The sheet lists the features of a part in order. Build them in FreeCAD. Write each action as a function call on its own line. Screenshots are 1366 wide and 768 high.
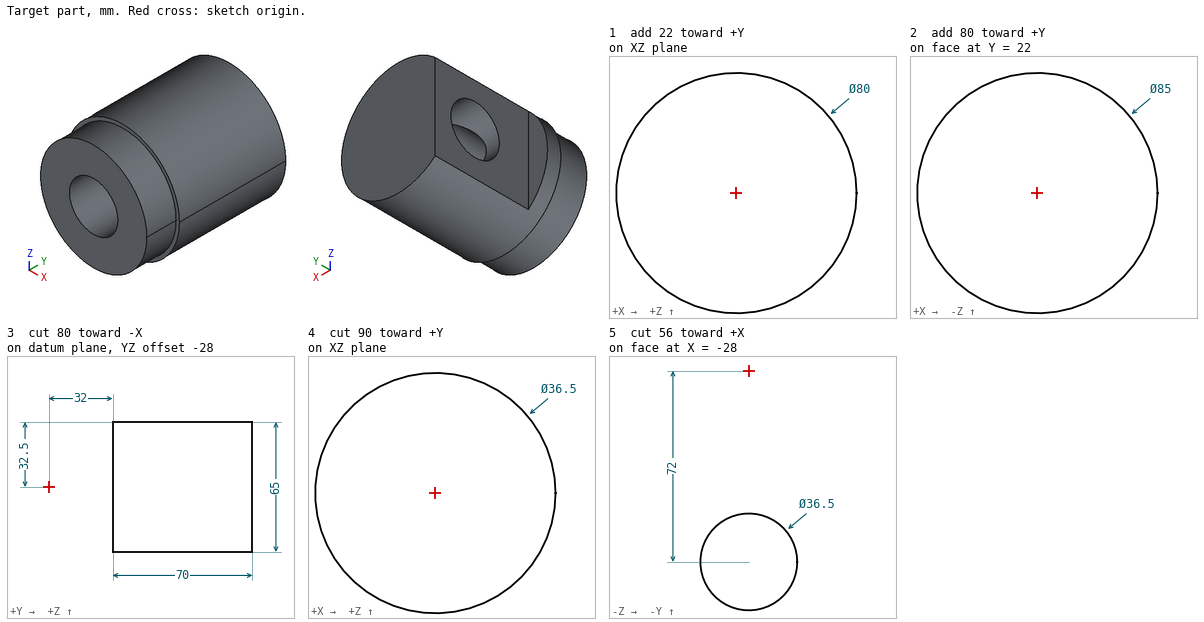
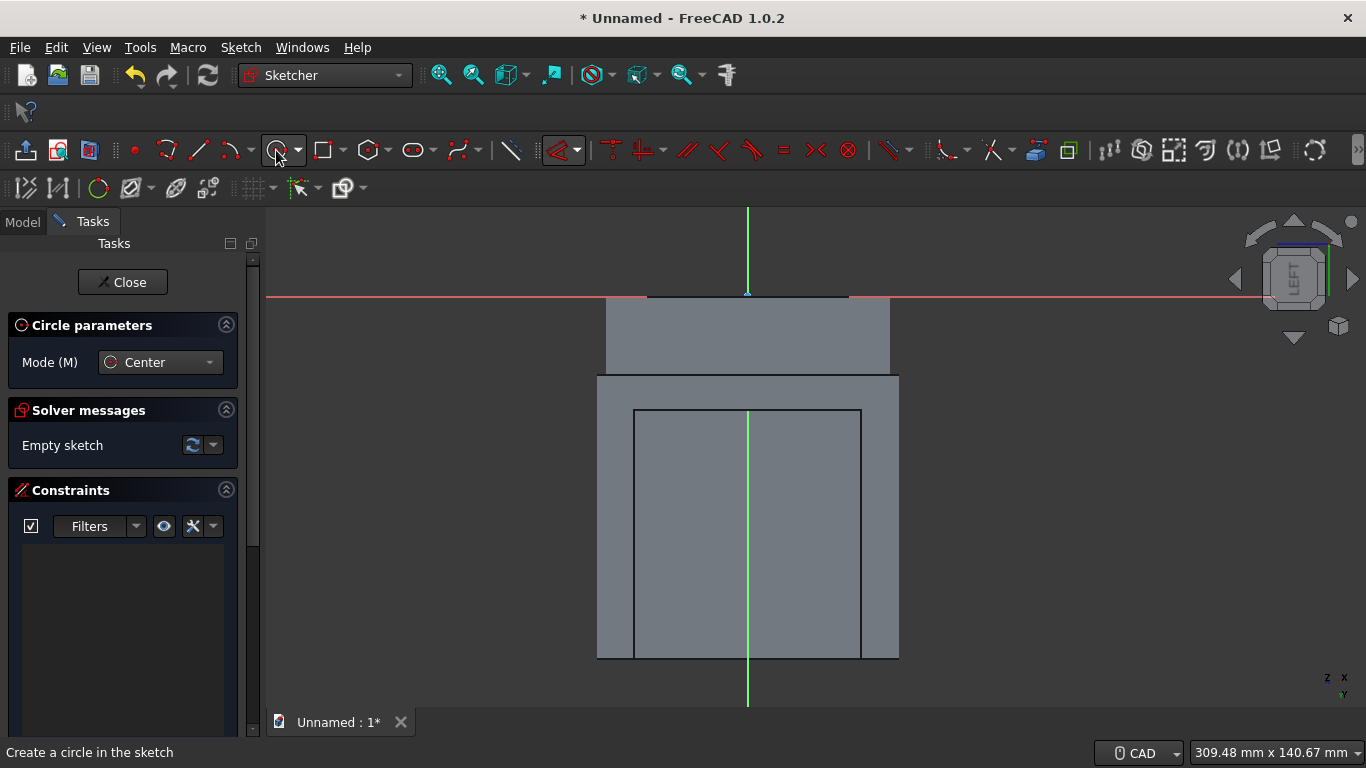
click(748, 553)
move(794, 507)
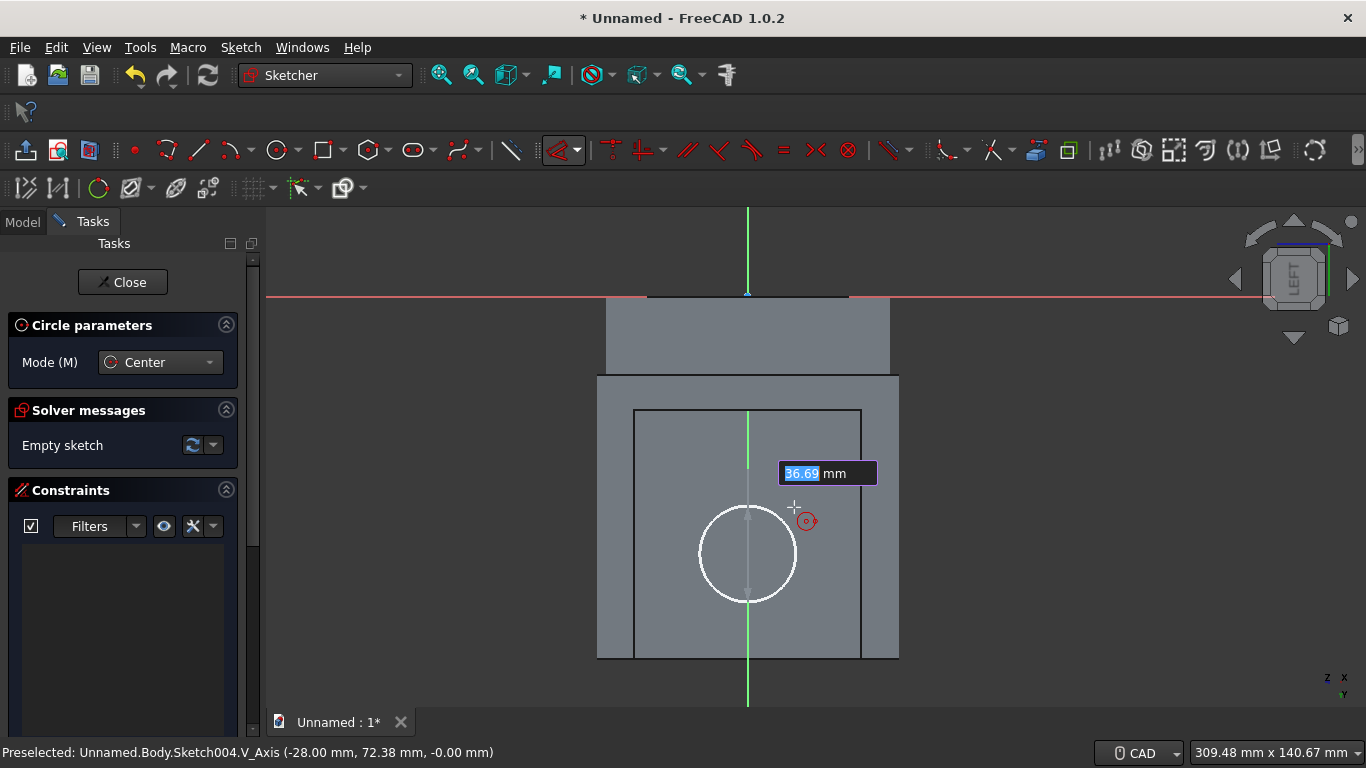
text(36.5)
key(Return)
key(Escape)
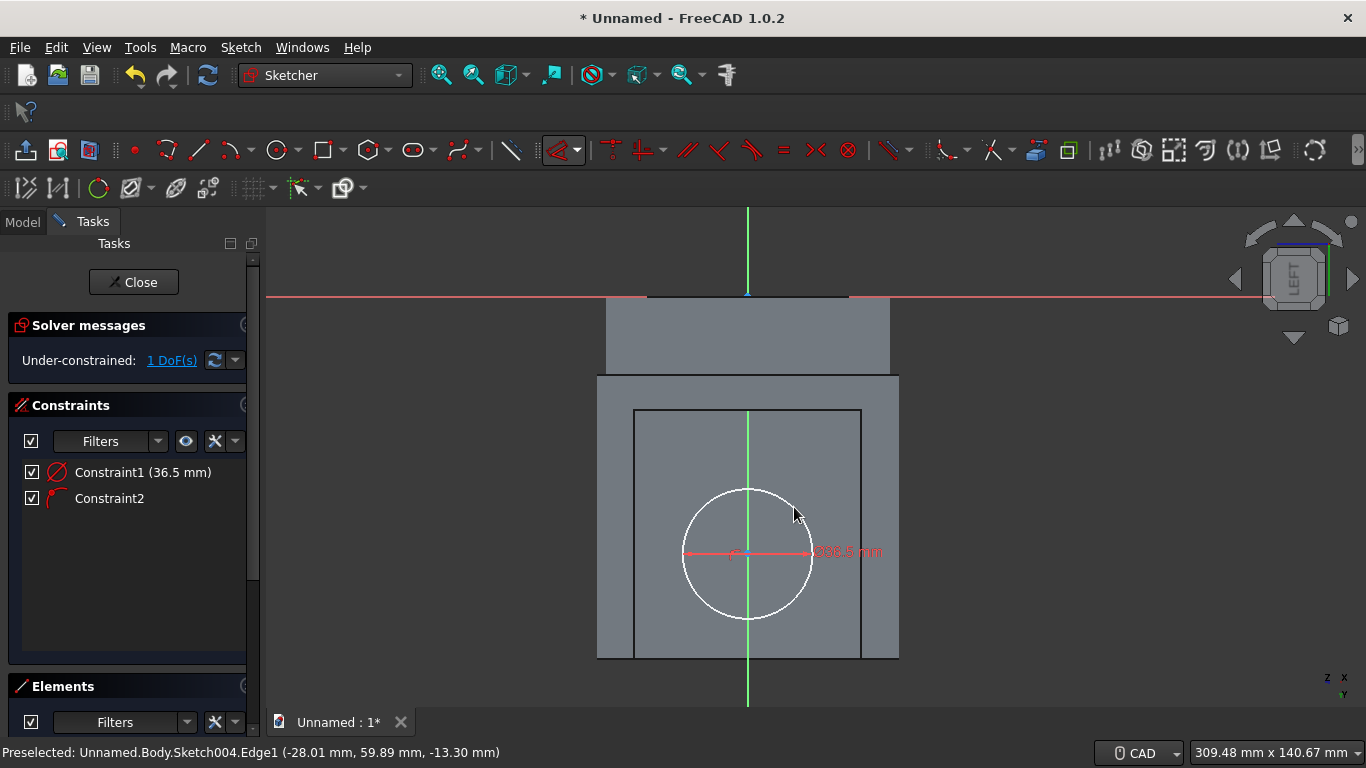
click(748, 554)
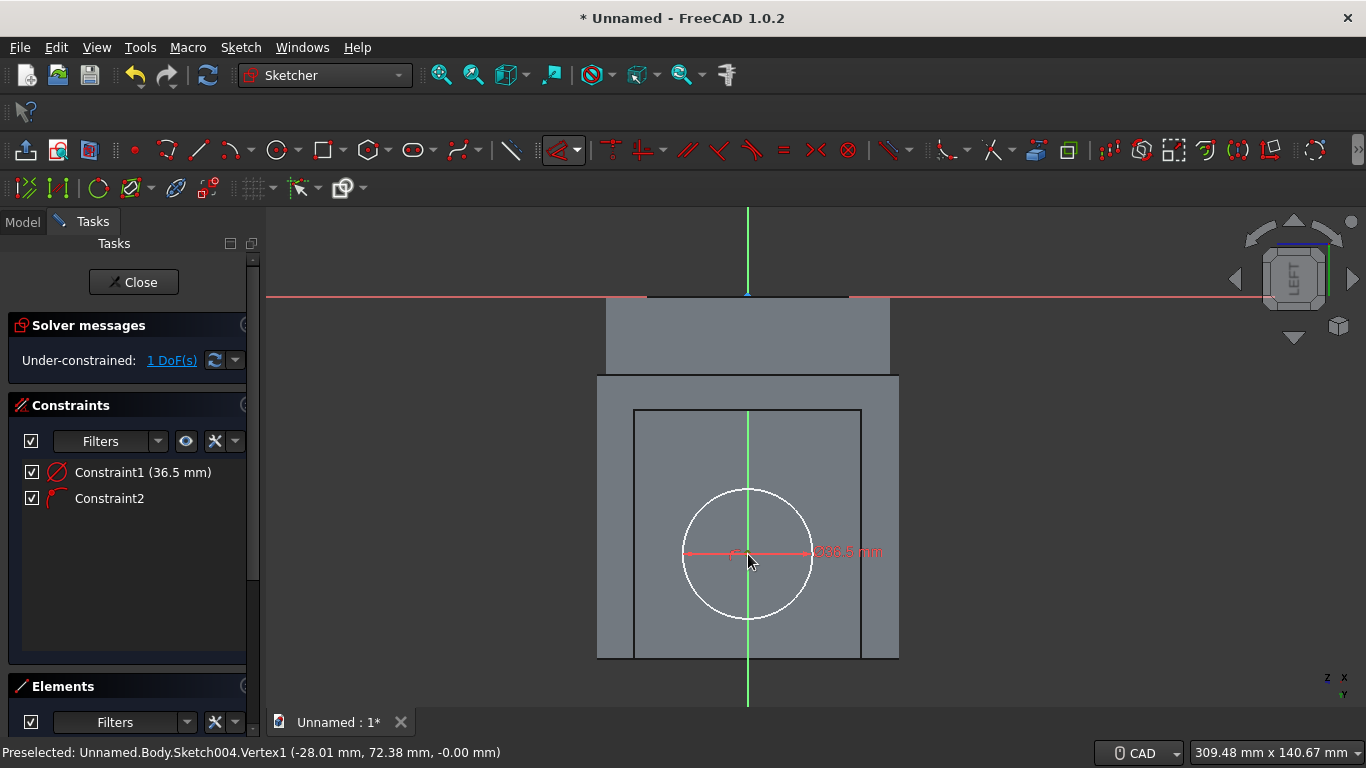
click(580, 150)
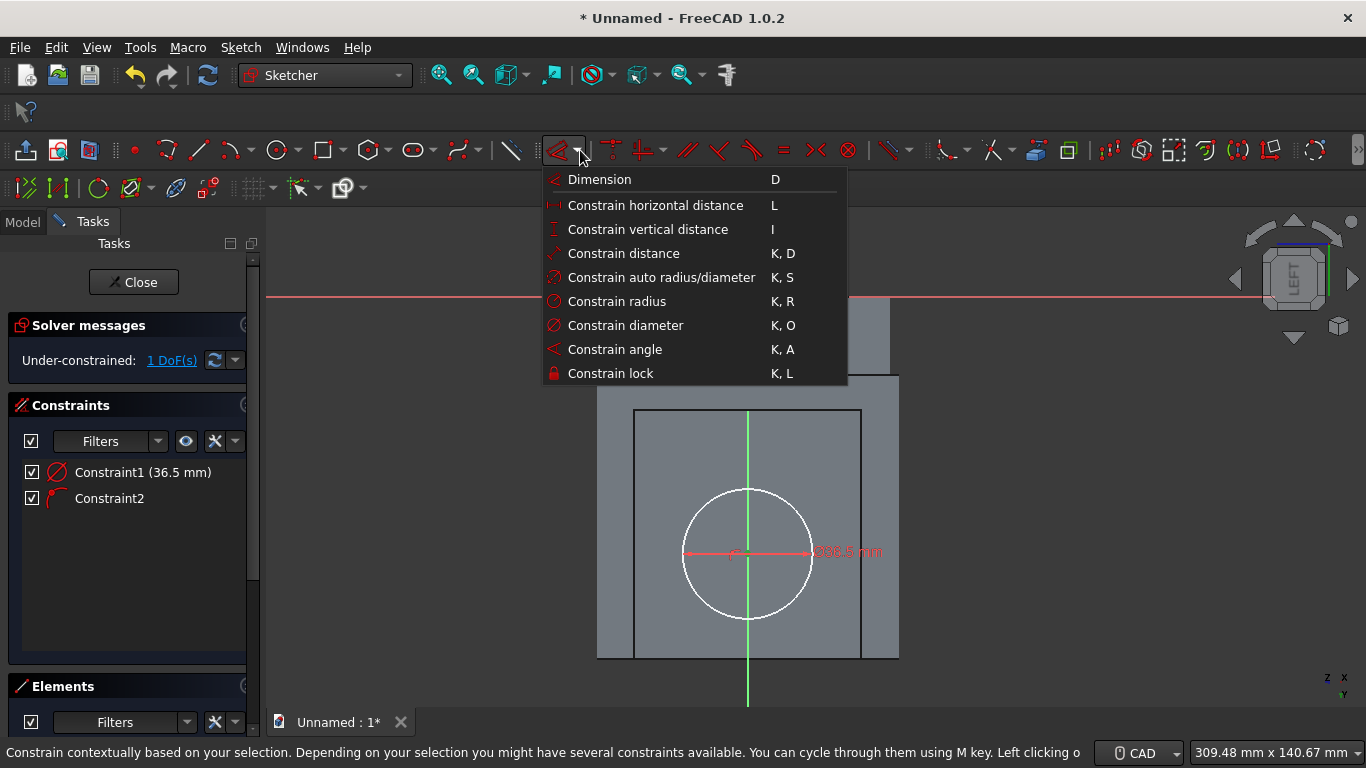
click(695, 229)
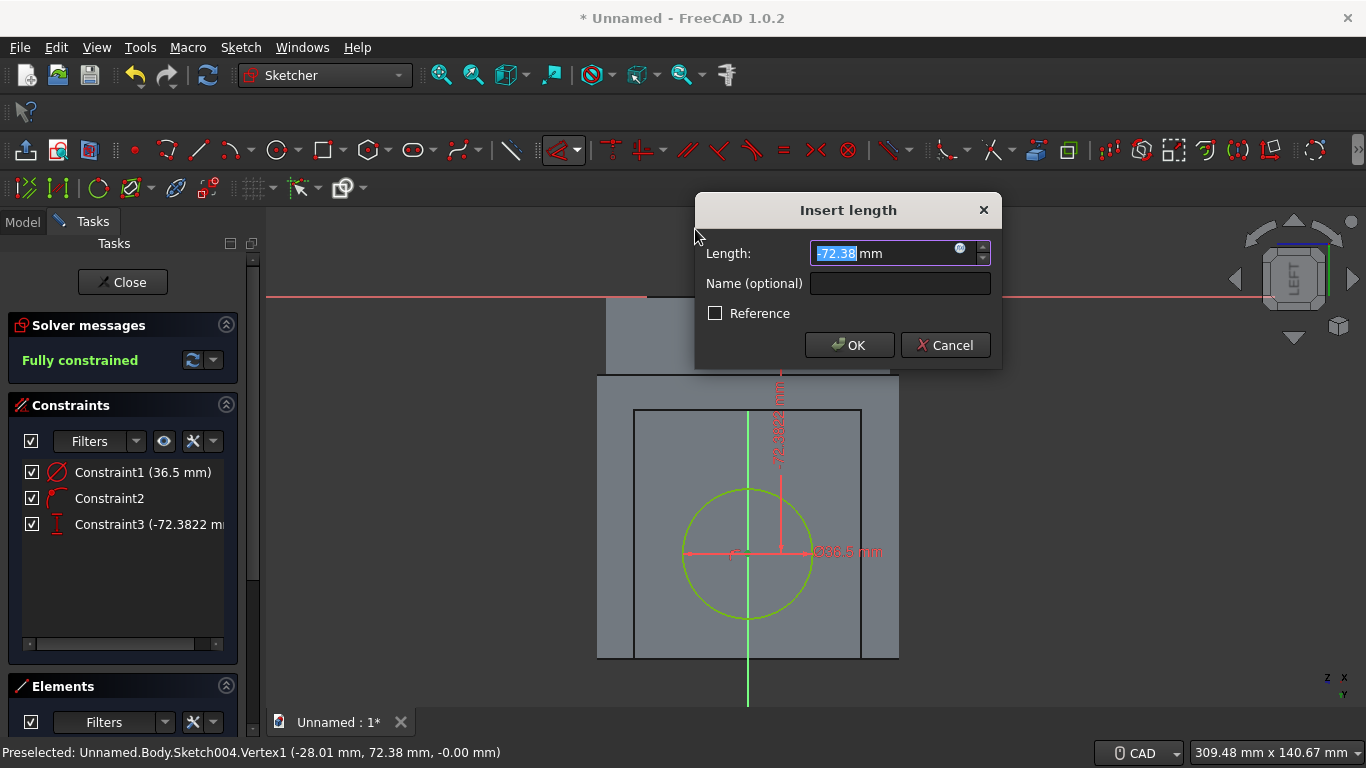
text(-72)
key(Return)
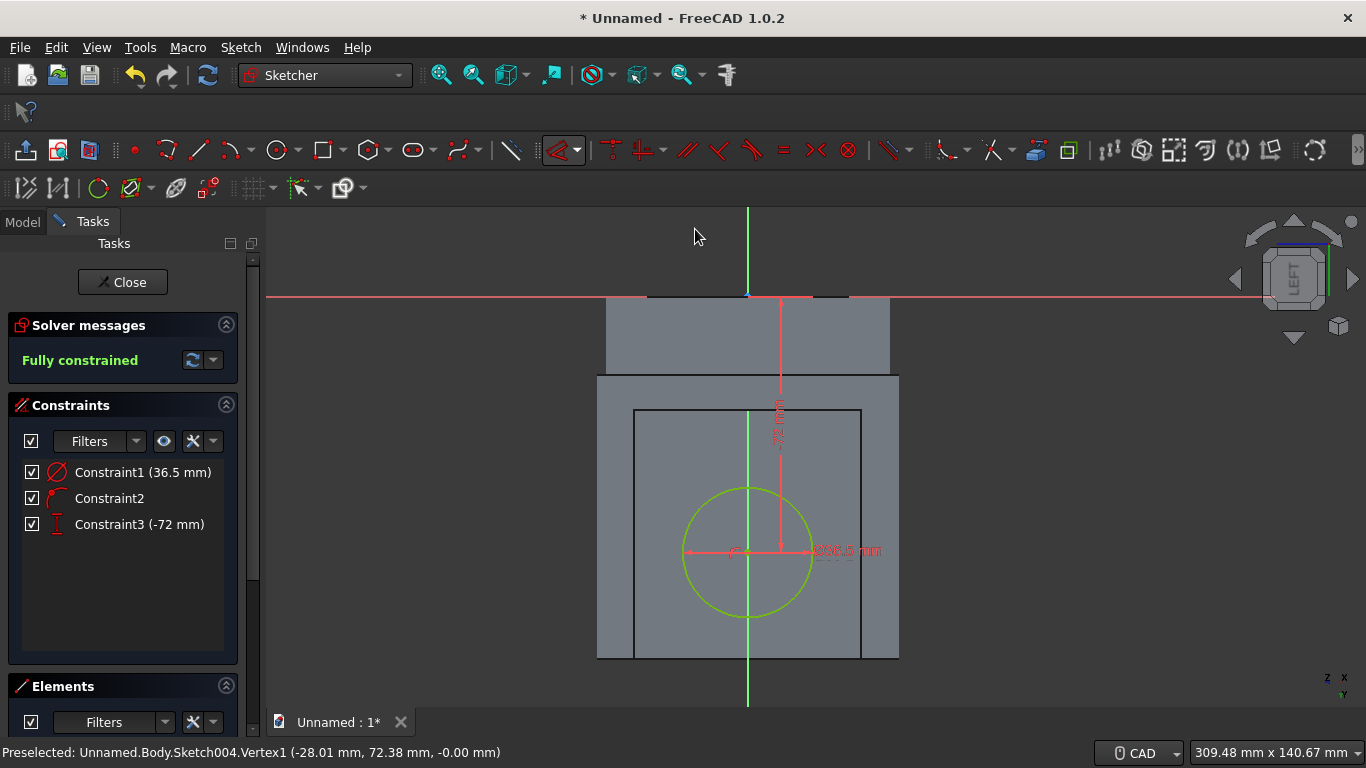
click(123, 282)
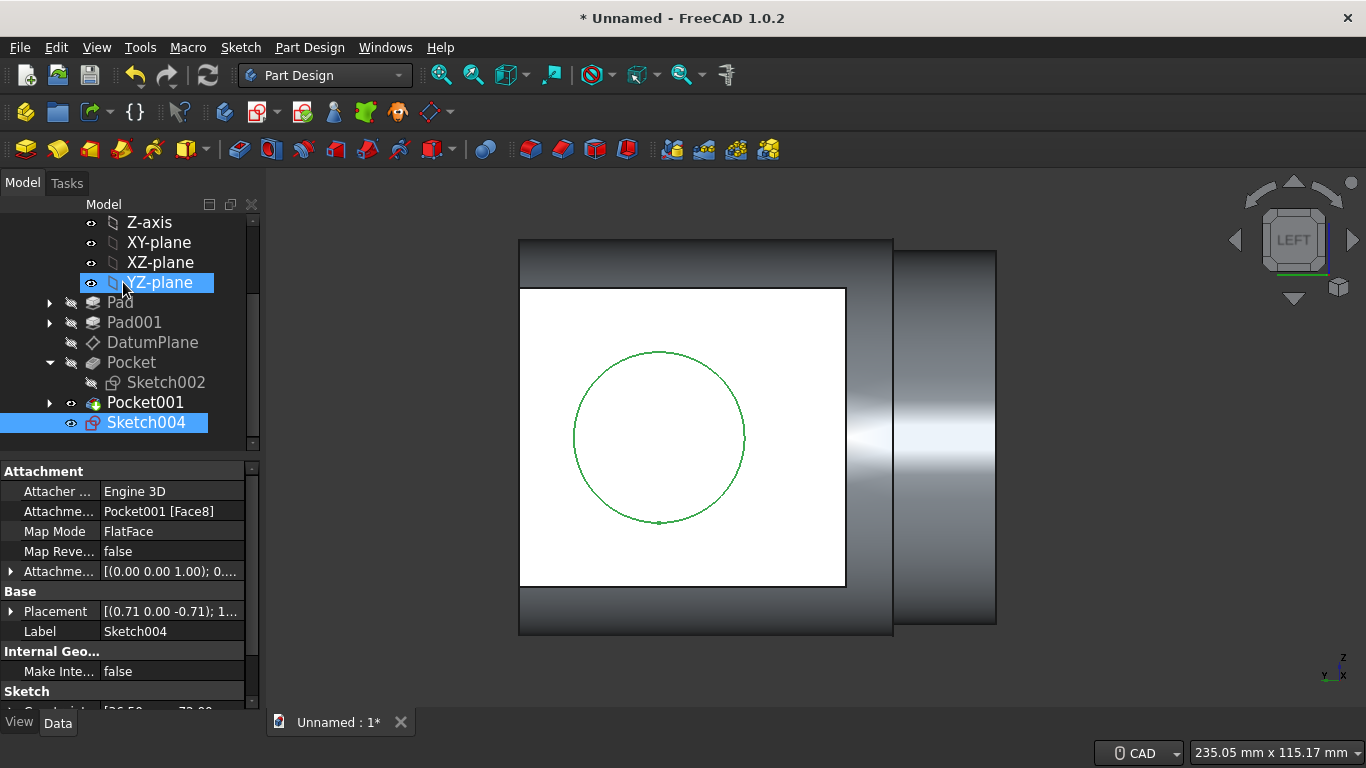
click(240, 150)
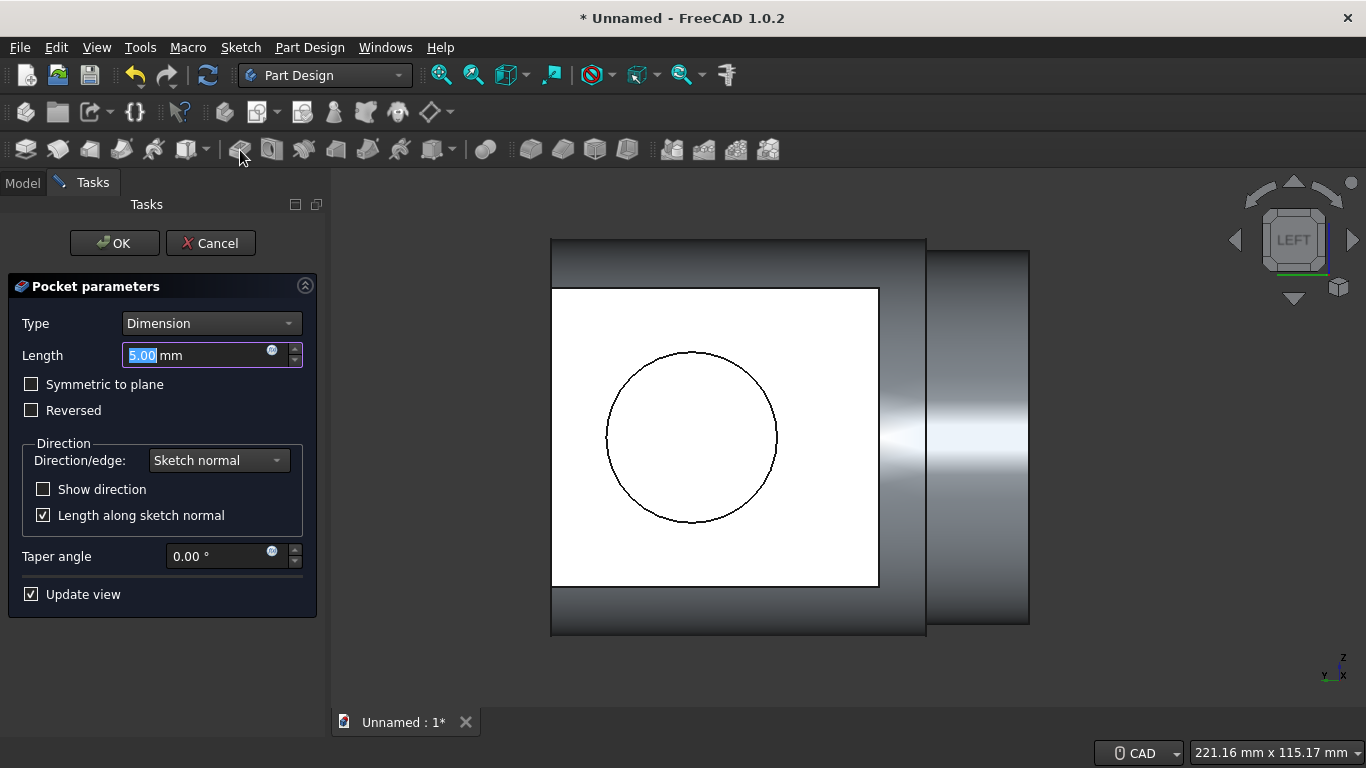
text(56)
key(Tab)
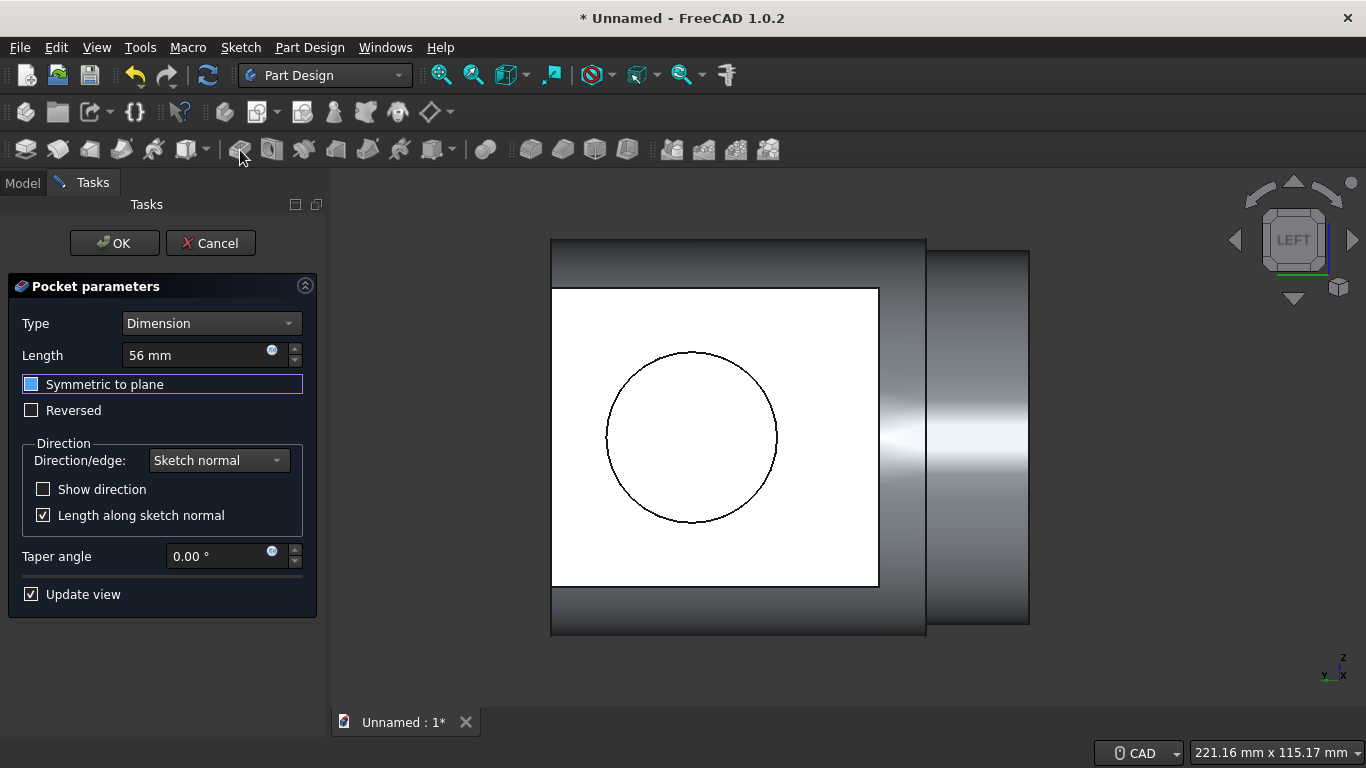
click(115, 243)